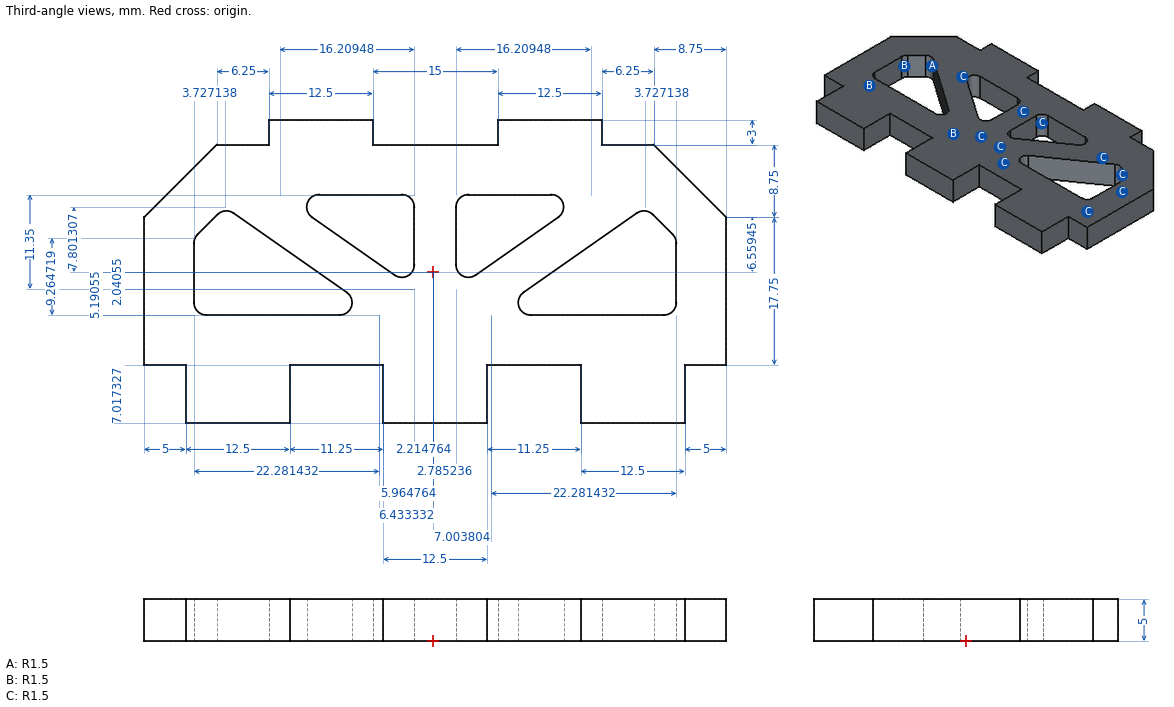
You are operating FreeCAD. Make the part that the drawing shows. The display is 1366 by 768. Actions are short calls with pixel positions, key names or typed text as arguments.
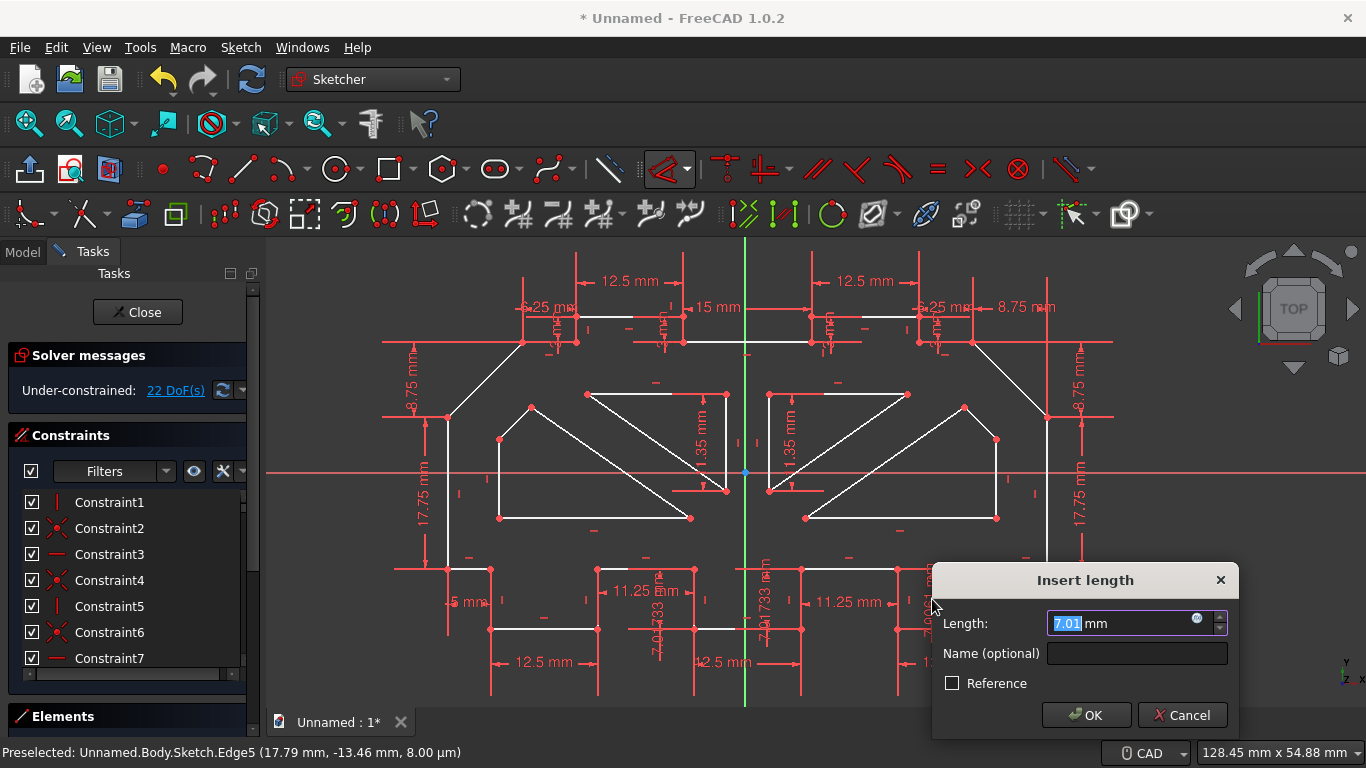
text(7.017327)
key(Return)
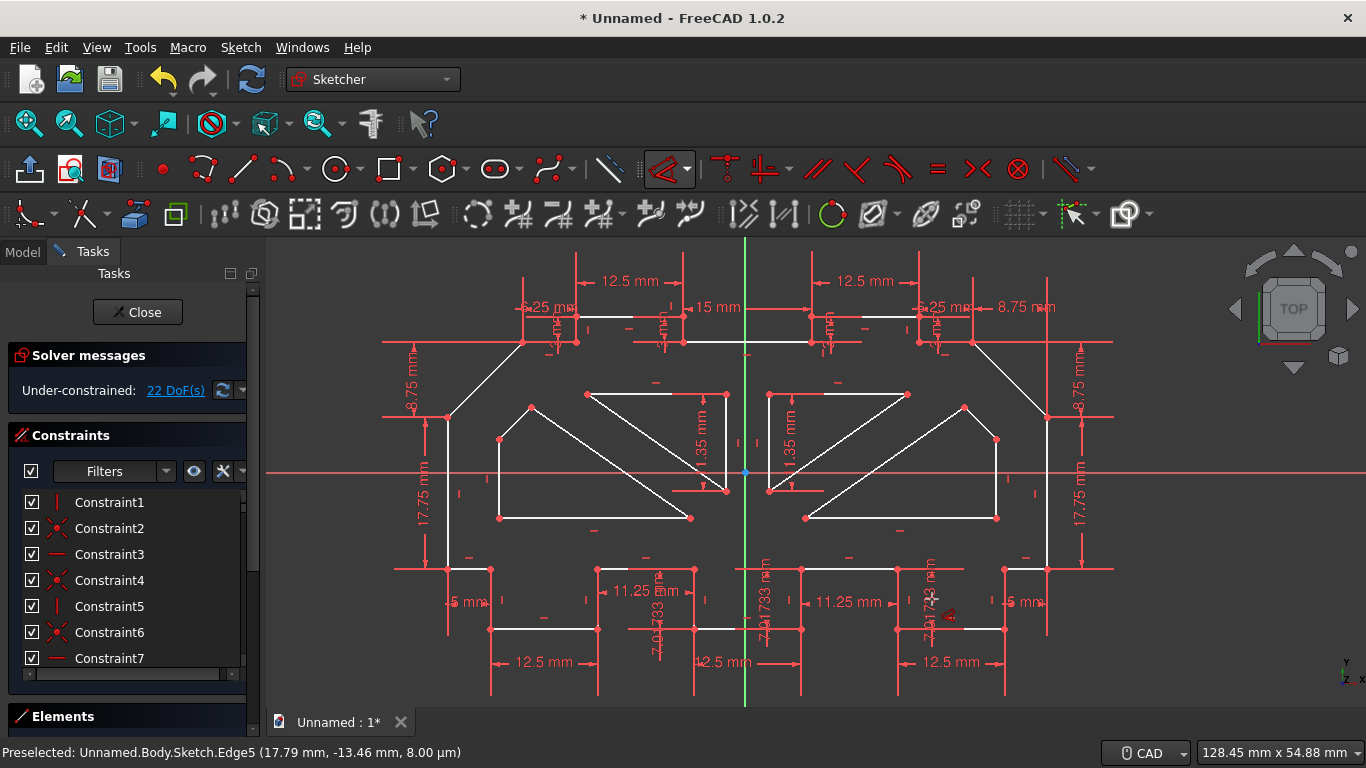
click(1005, 611)
click(971, 578)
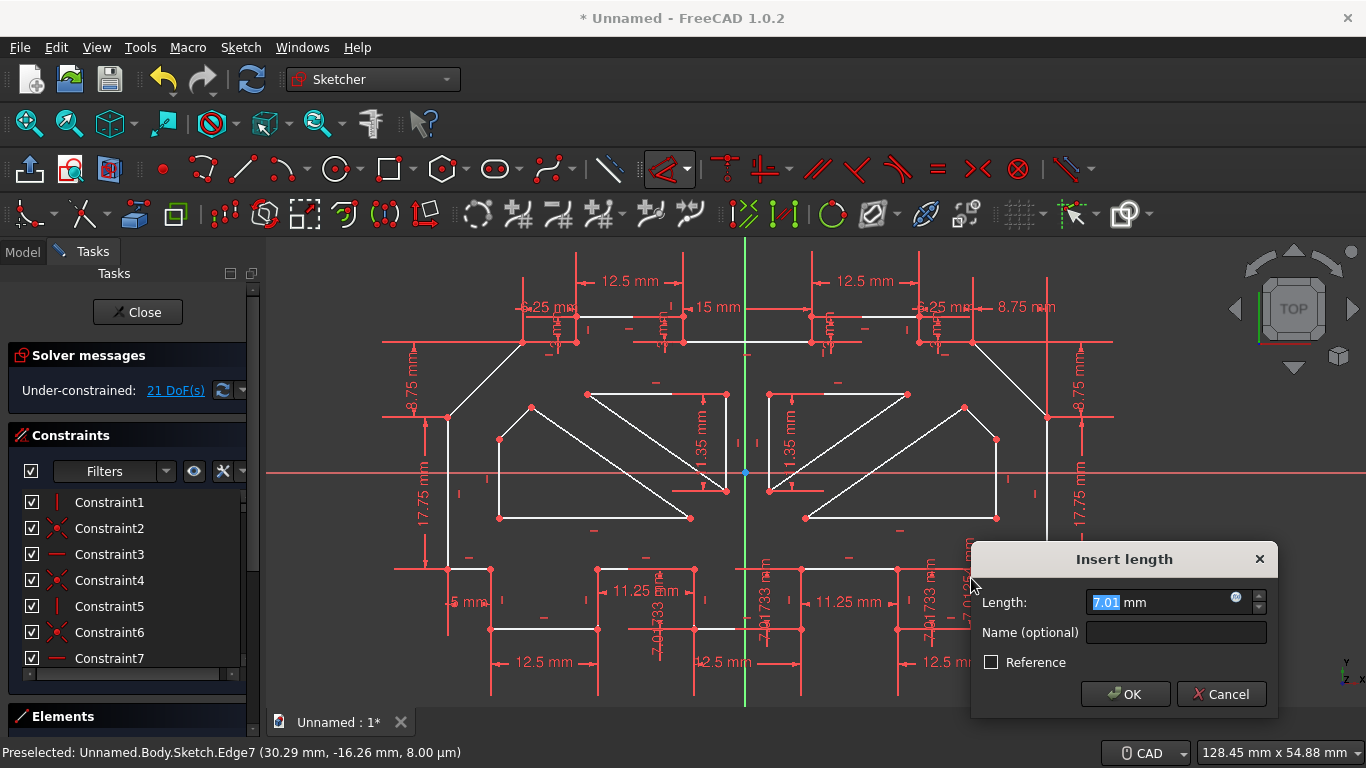
text(7.017327)
key(Return)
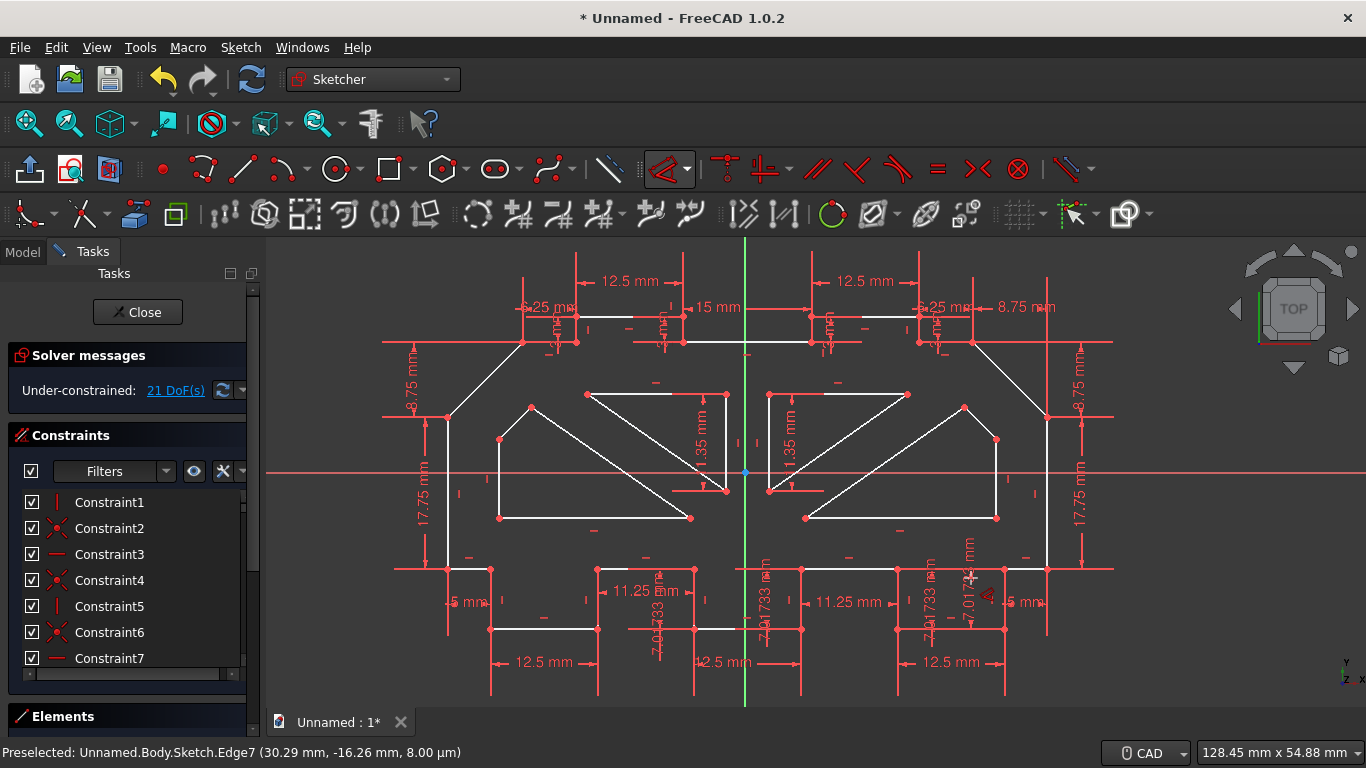
click(491, 587)
click(525, 578)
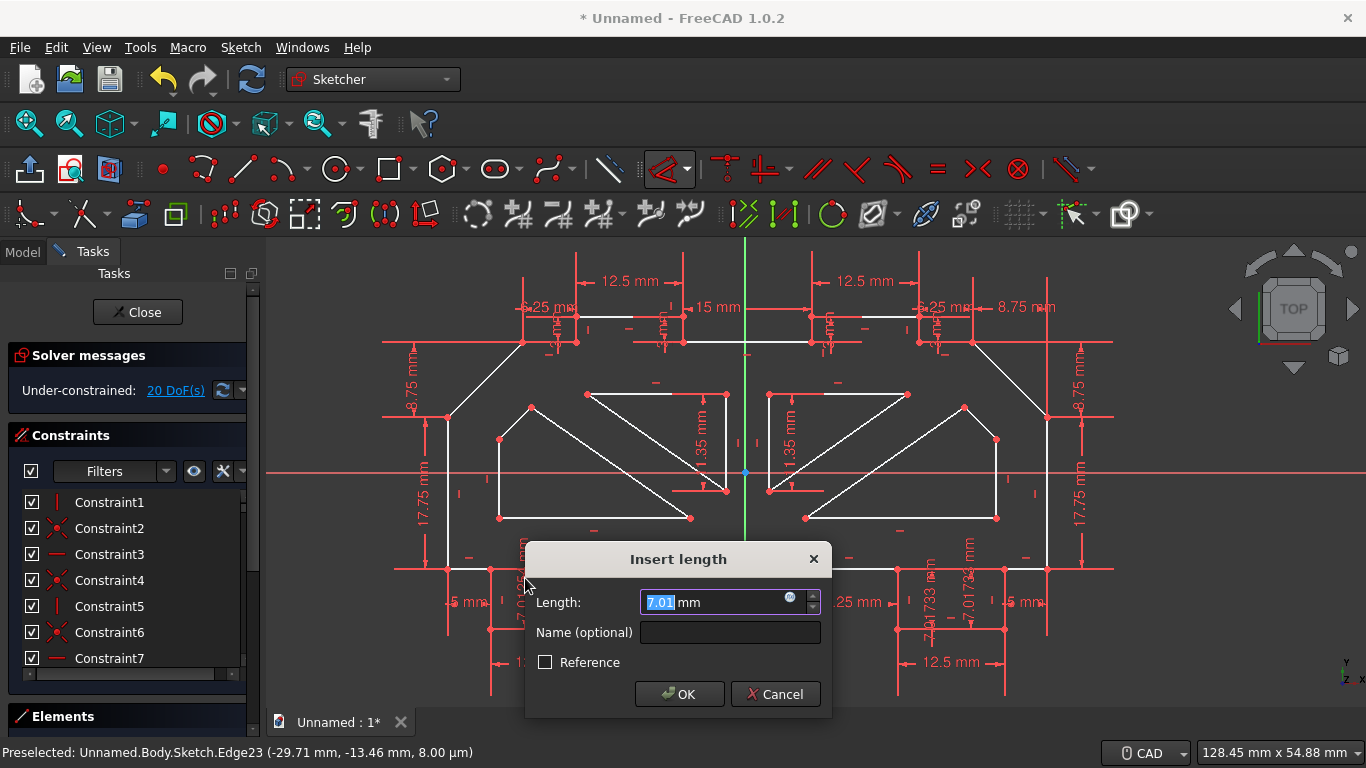
text(7.017327)
key(Return)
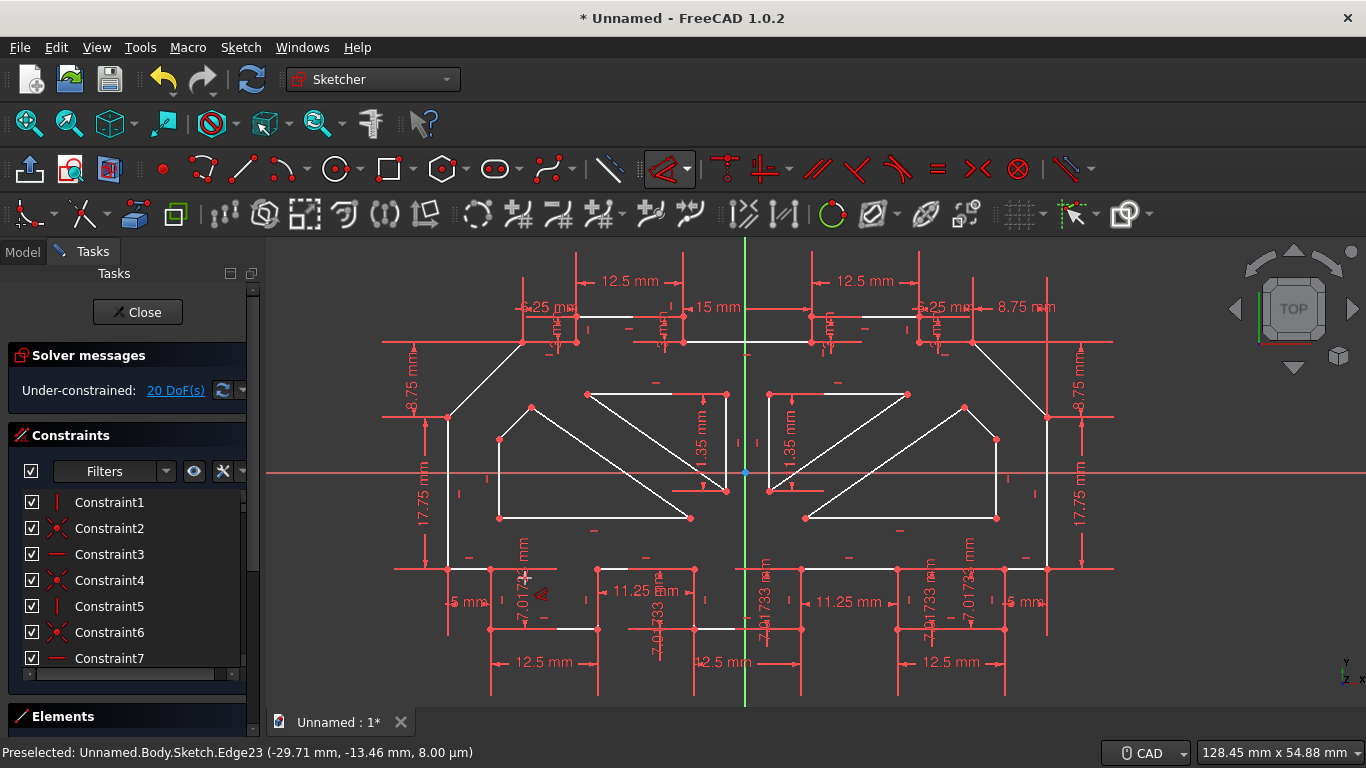
click(499, 495)
click(465, 451)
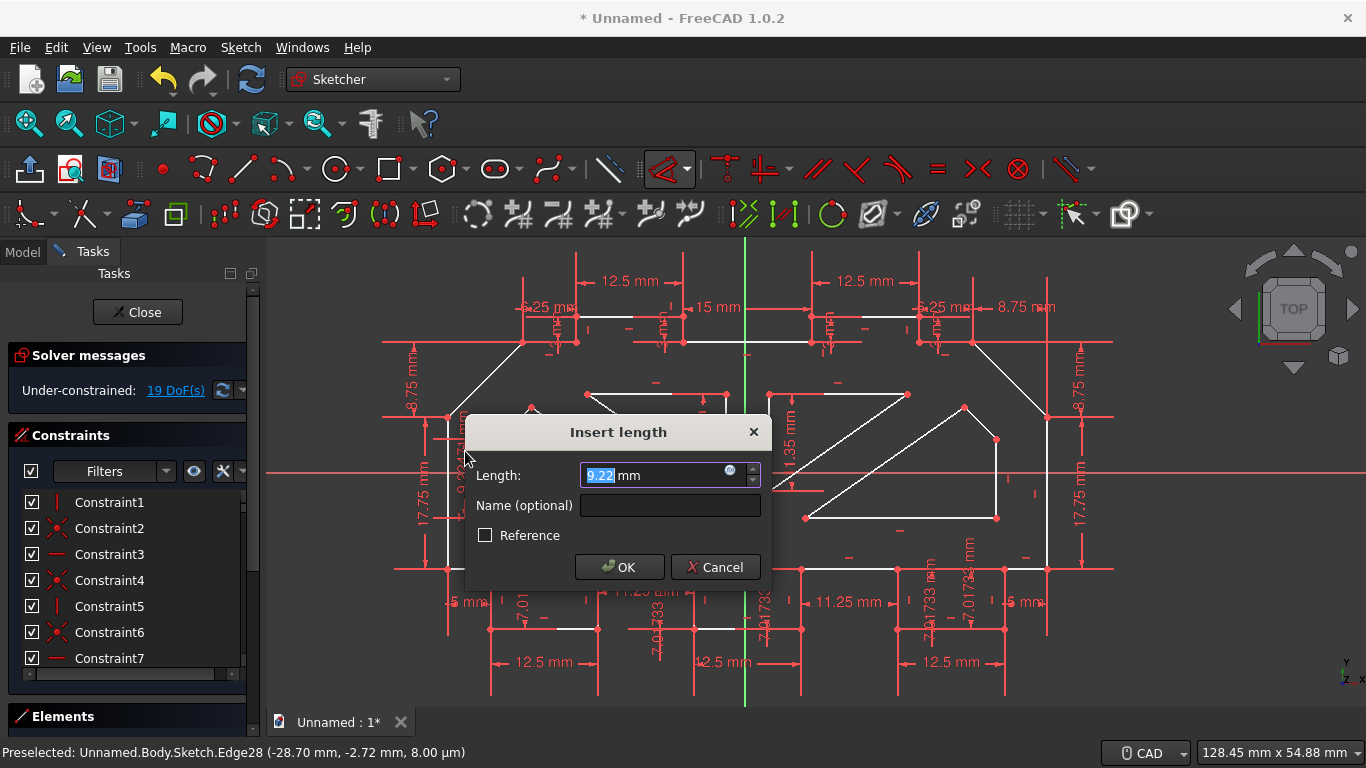
text(9.264719)
key(Return)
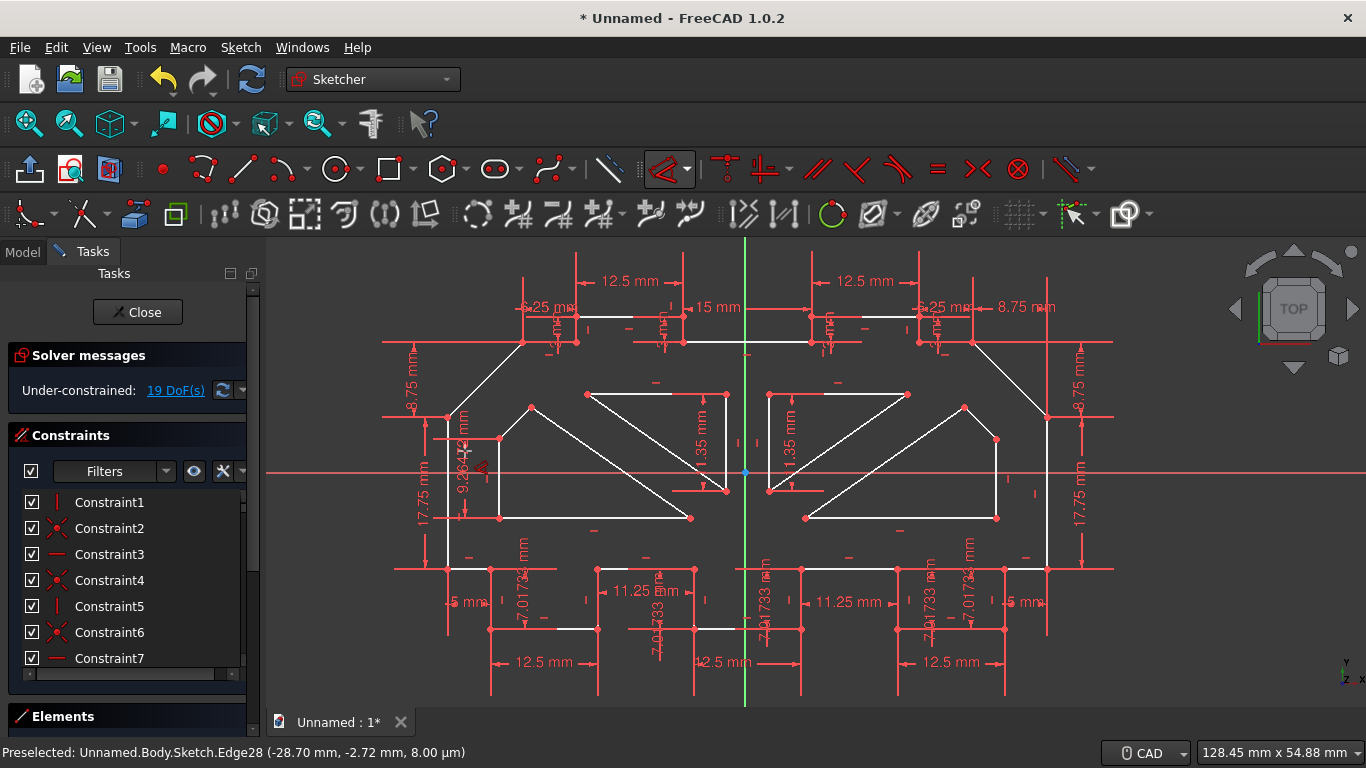
scroll(996, 463, up, 2)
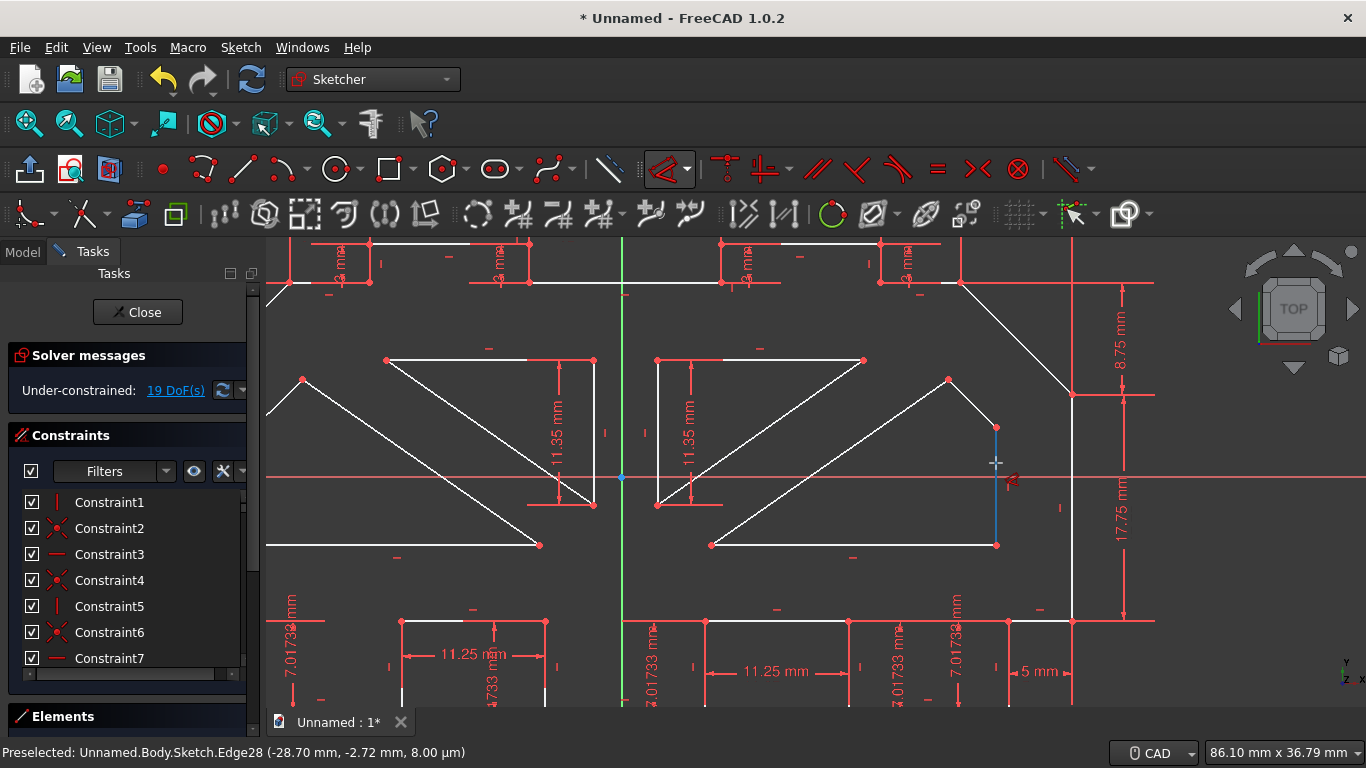
click(996, 463)
click(1030, 459)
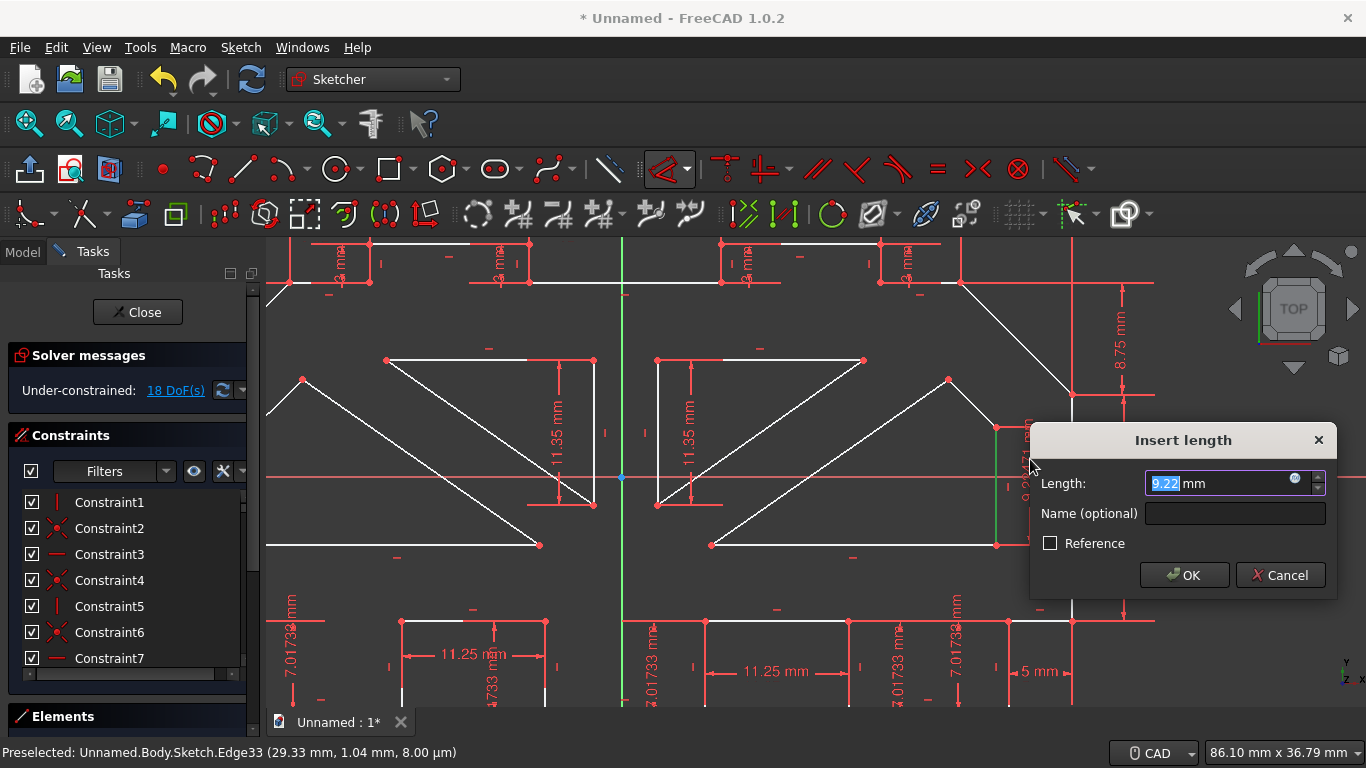
text(9.264719)
key(Return)